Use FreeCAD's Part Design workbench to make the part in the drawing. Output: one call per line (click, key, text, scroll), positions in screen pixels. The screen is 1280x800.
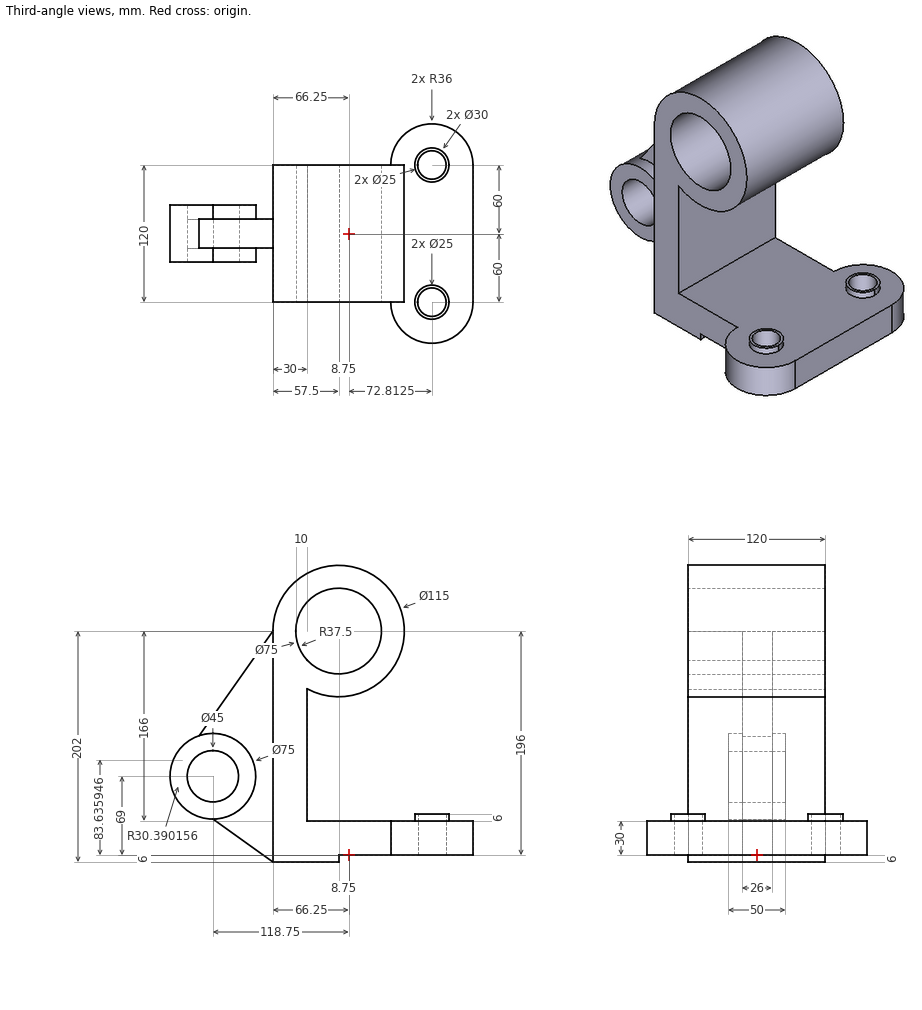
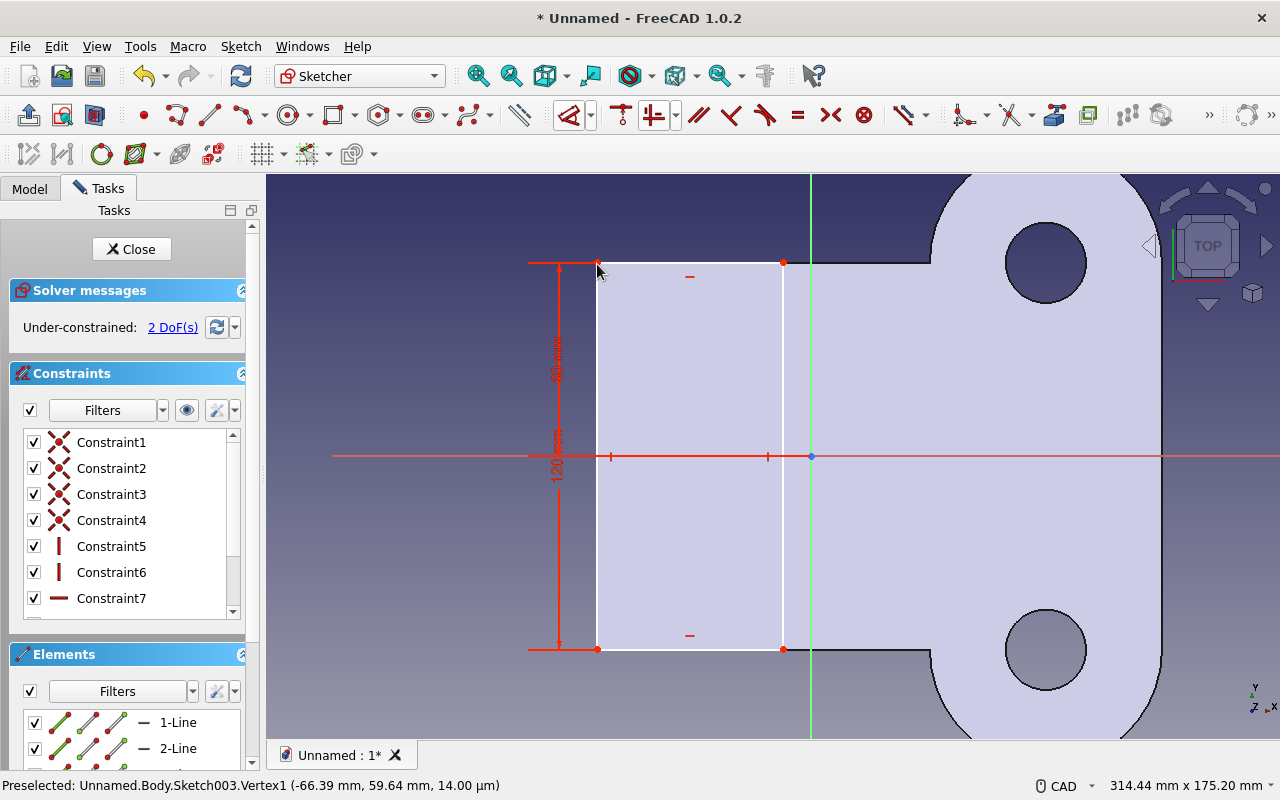
click(653, 650)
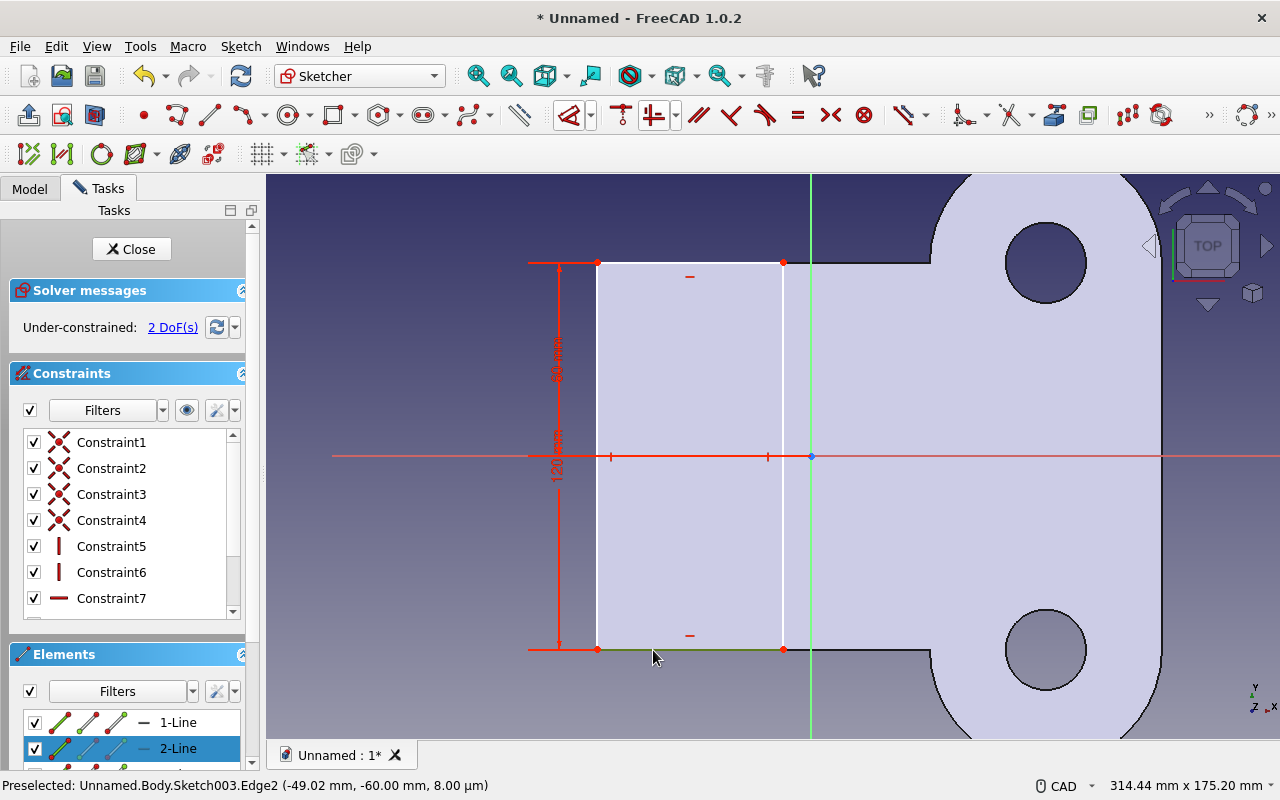
key(l)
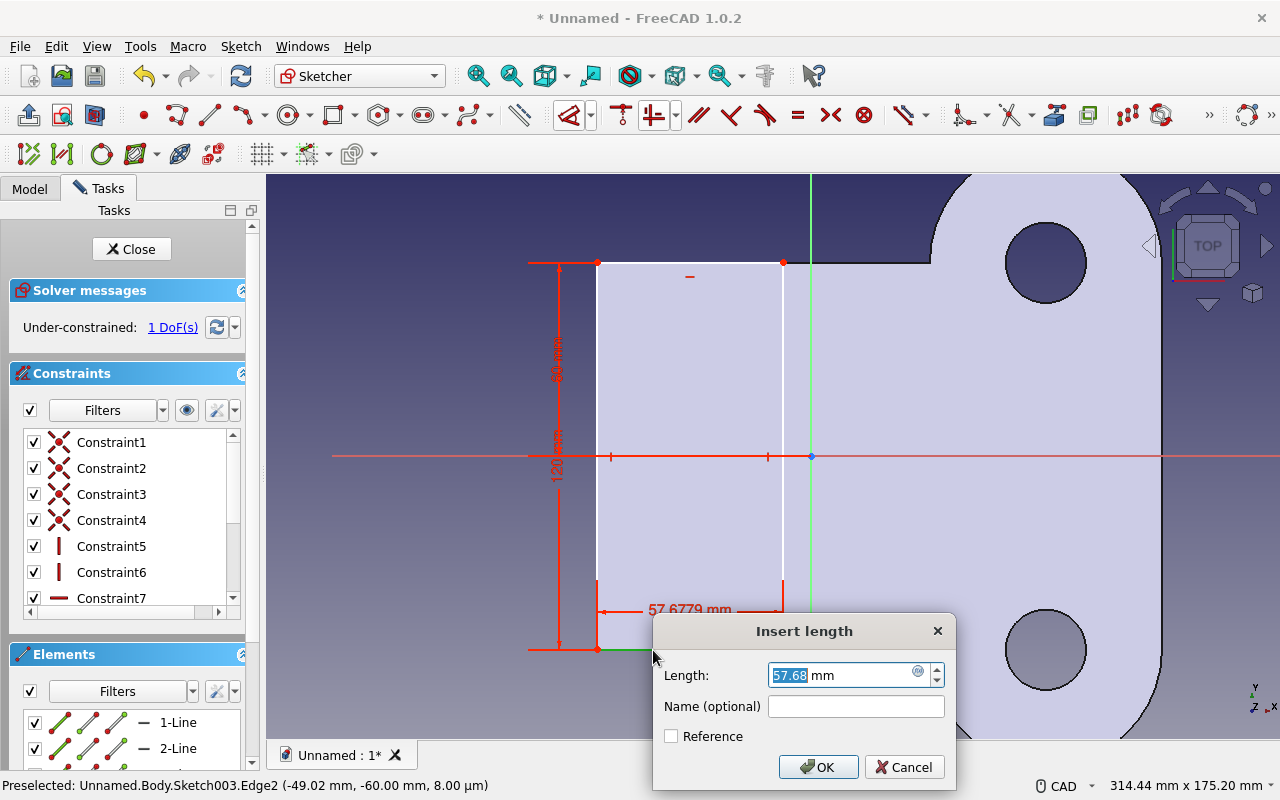
text(57.5)
key(Return)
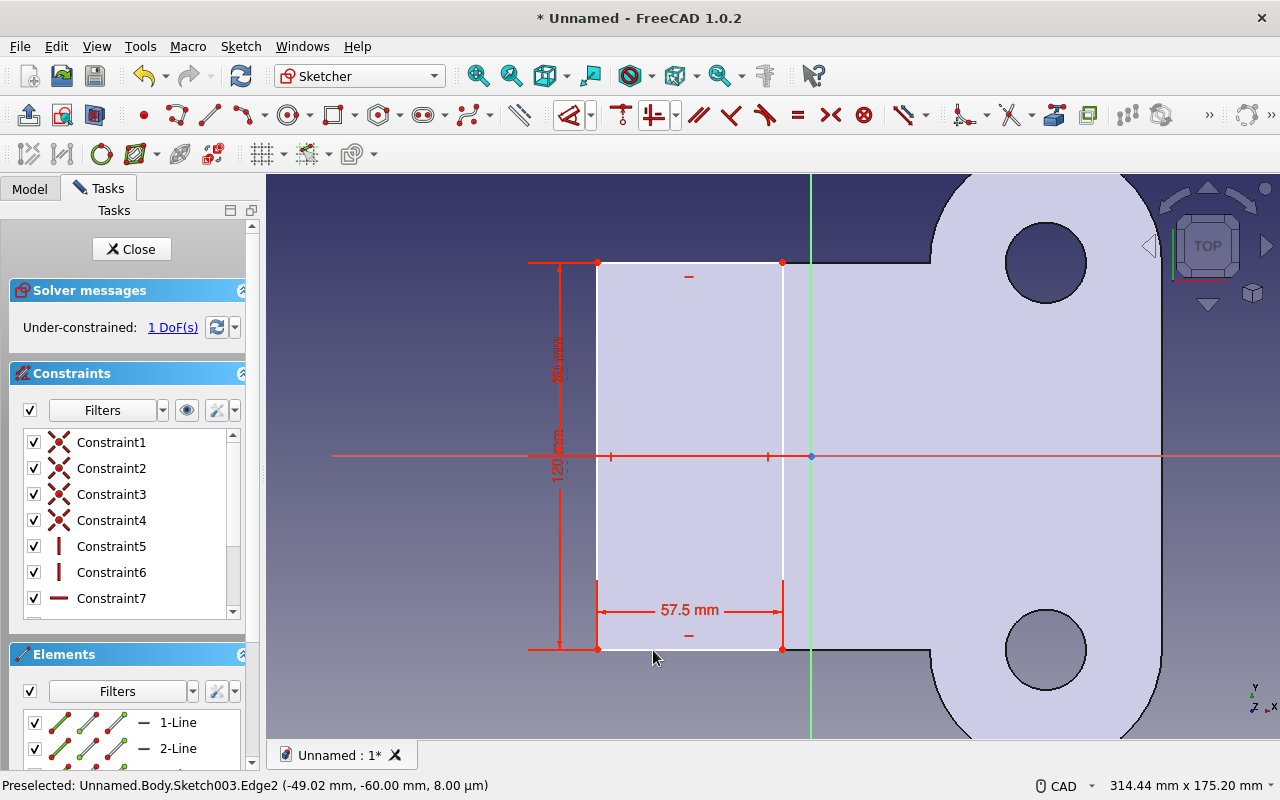
scroll(783, 650, up, 2)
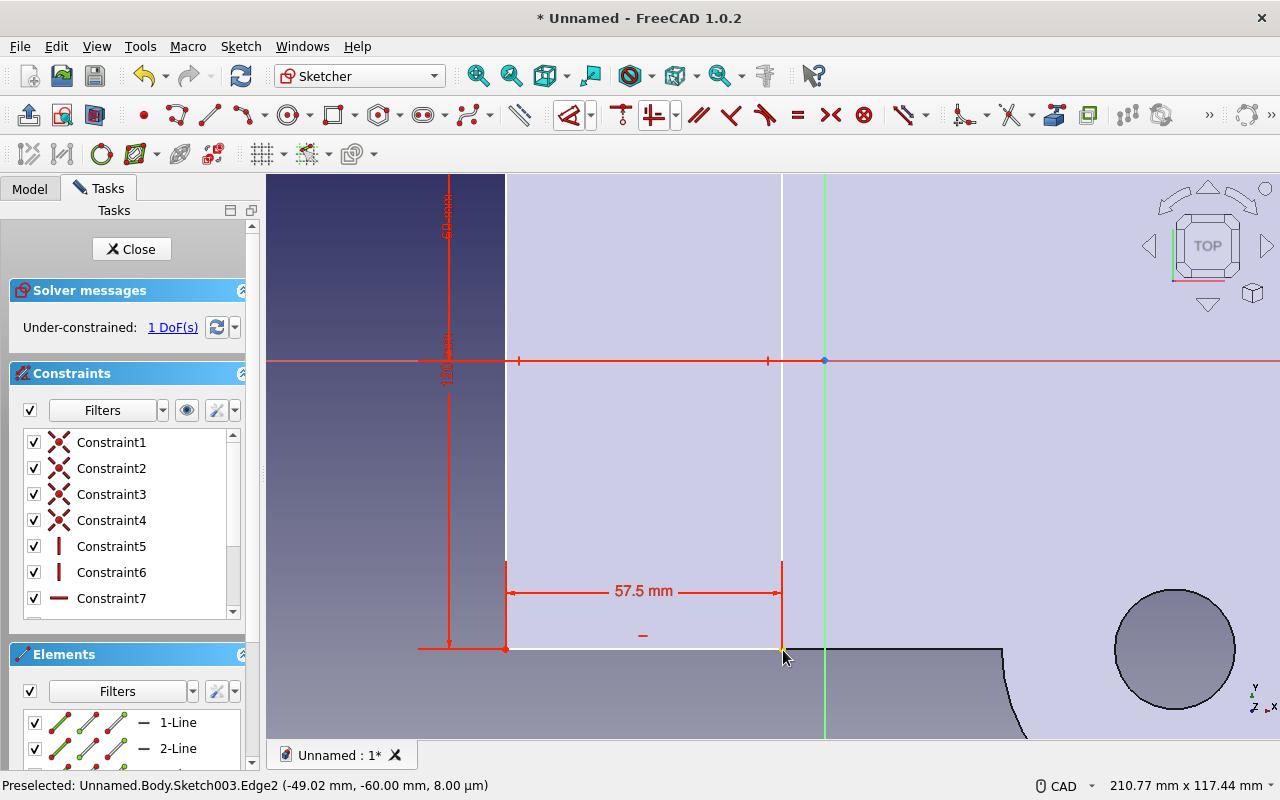
click(782, 649)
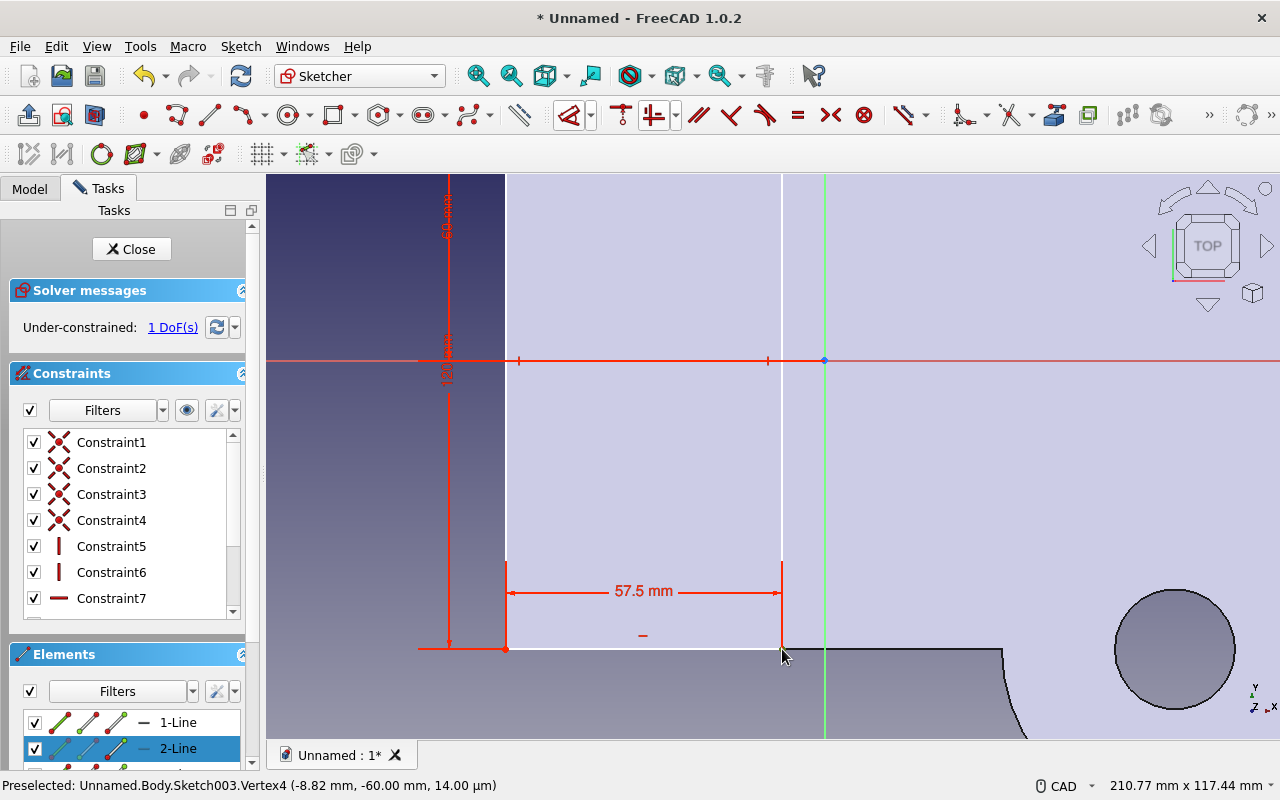
key(l)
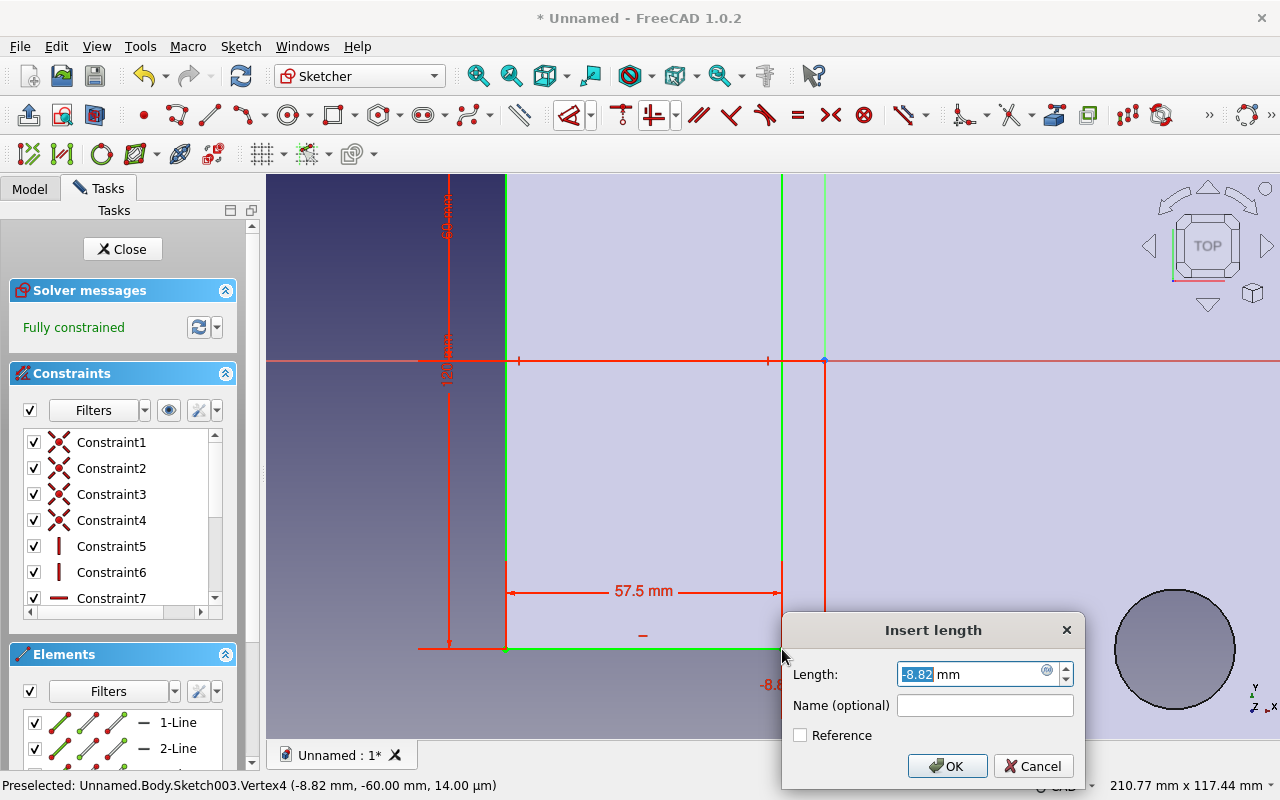
text(-8.75)
key(Return)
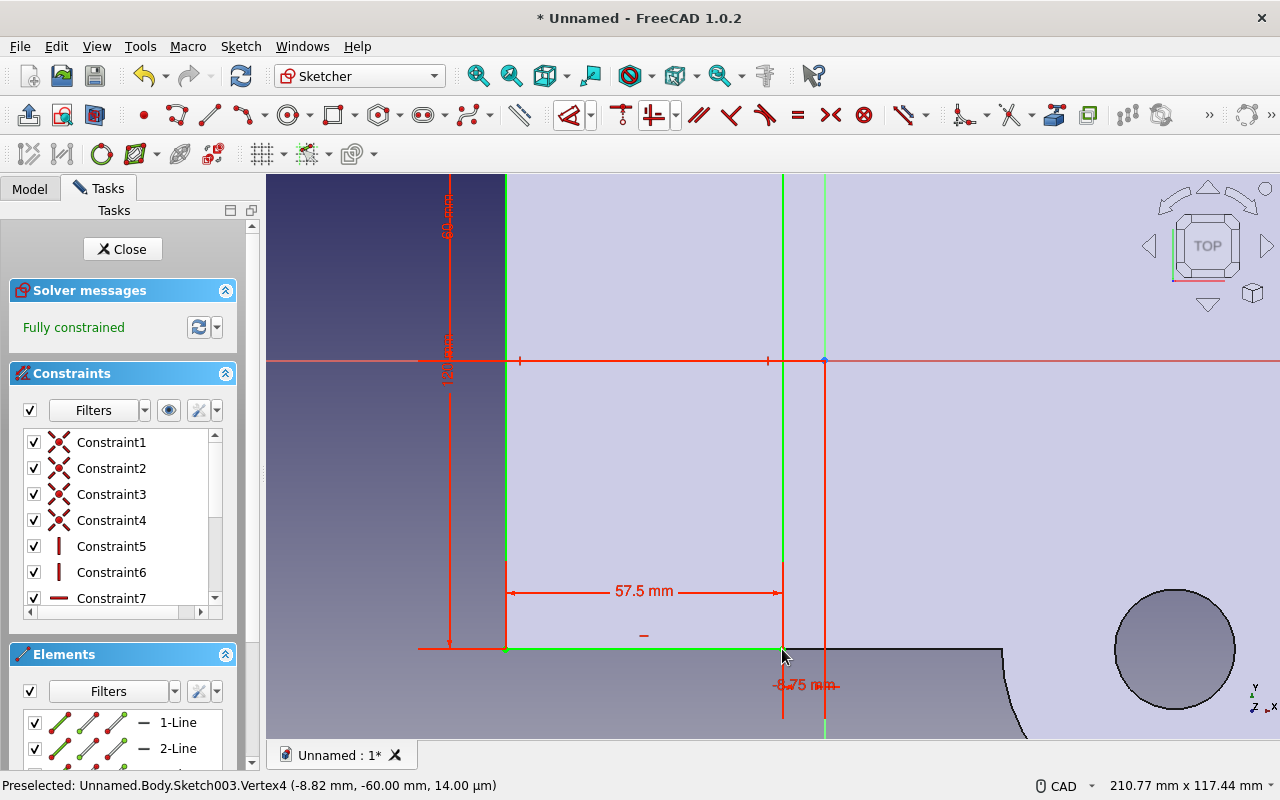
click(123, 249)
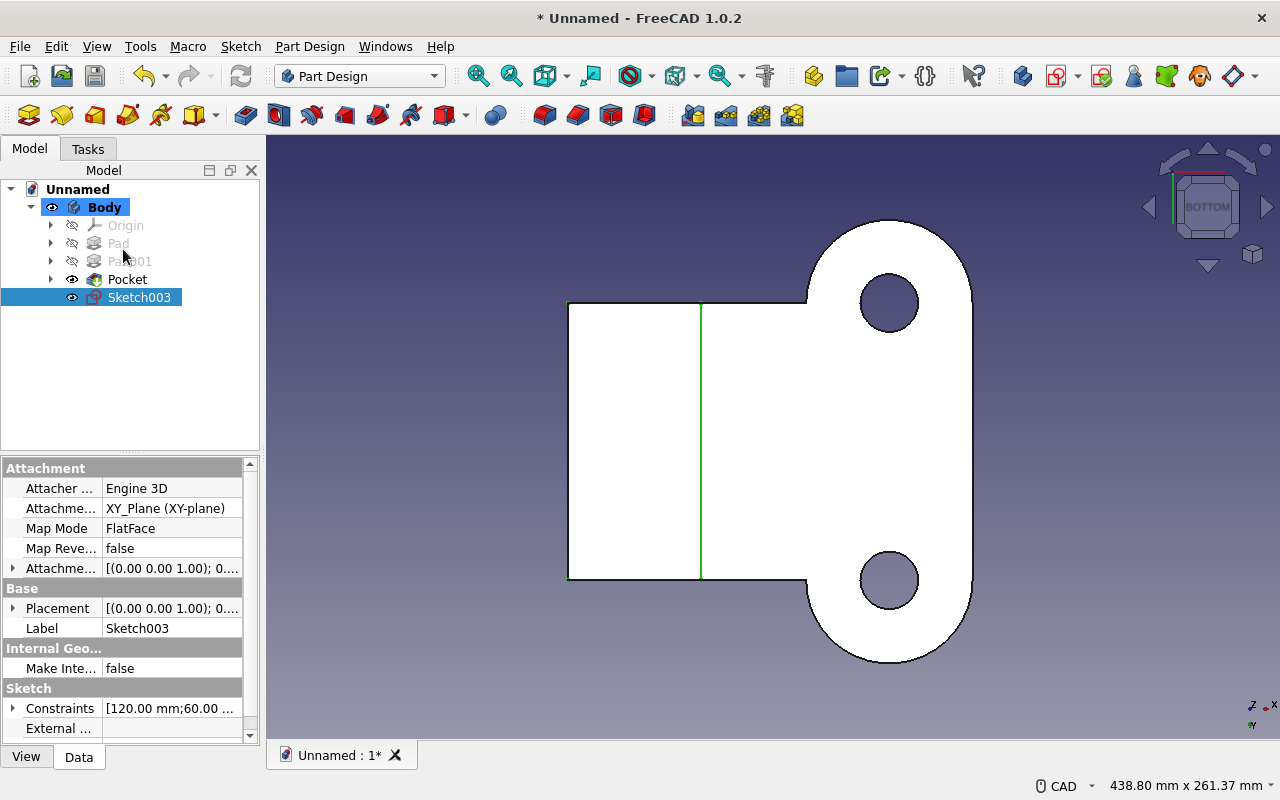
click(29, 116)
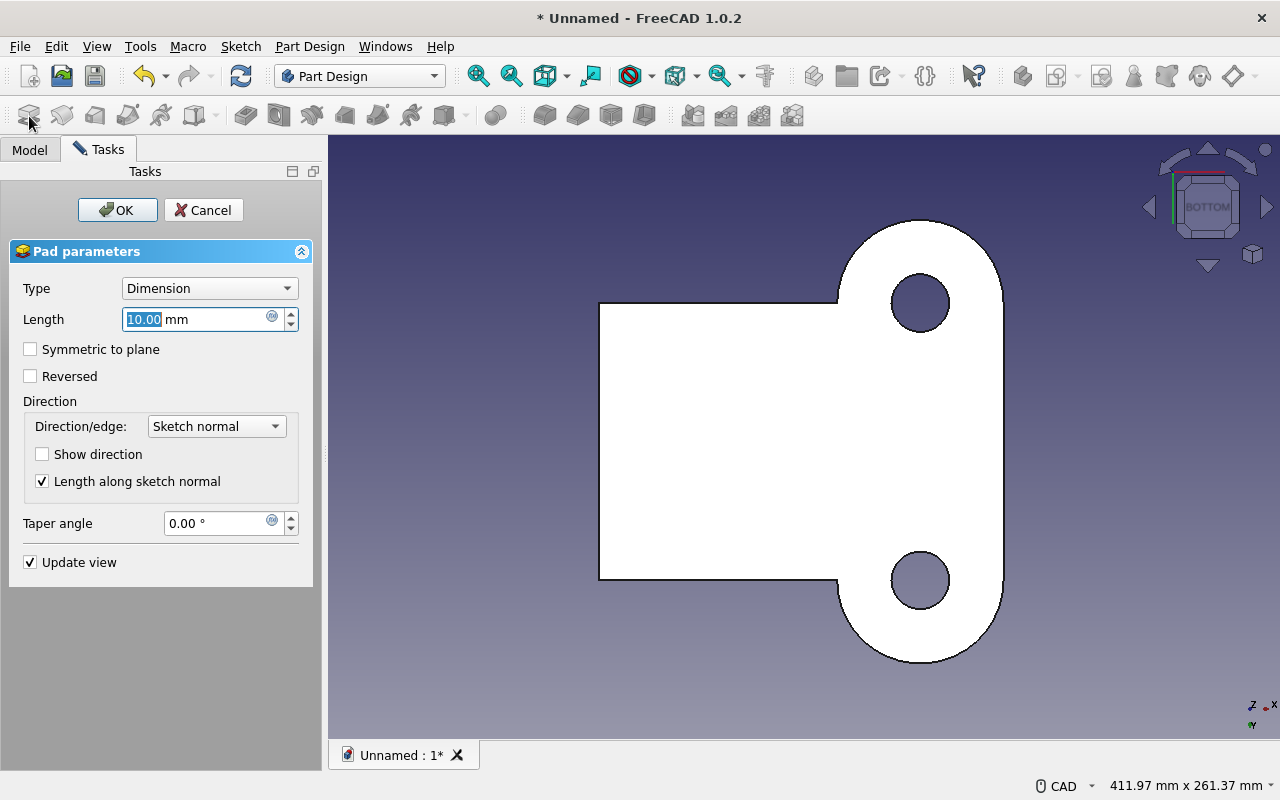
text(6)
key(Tab)